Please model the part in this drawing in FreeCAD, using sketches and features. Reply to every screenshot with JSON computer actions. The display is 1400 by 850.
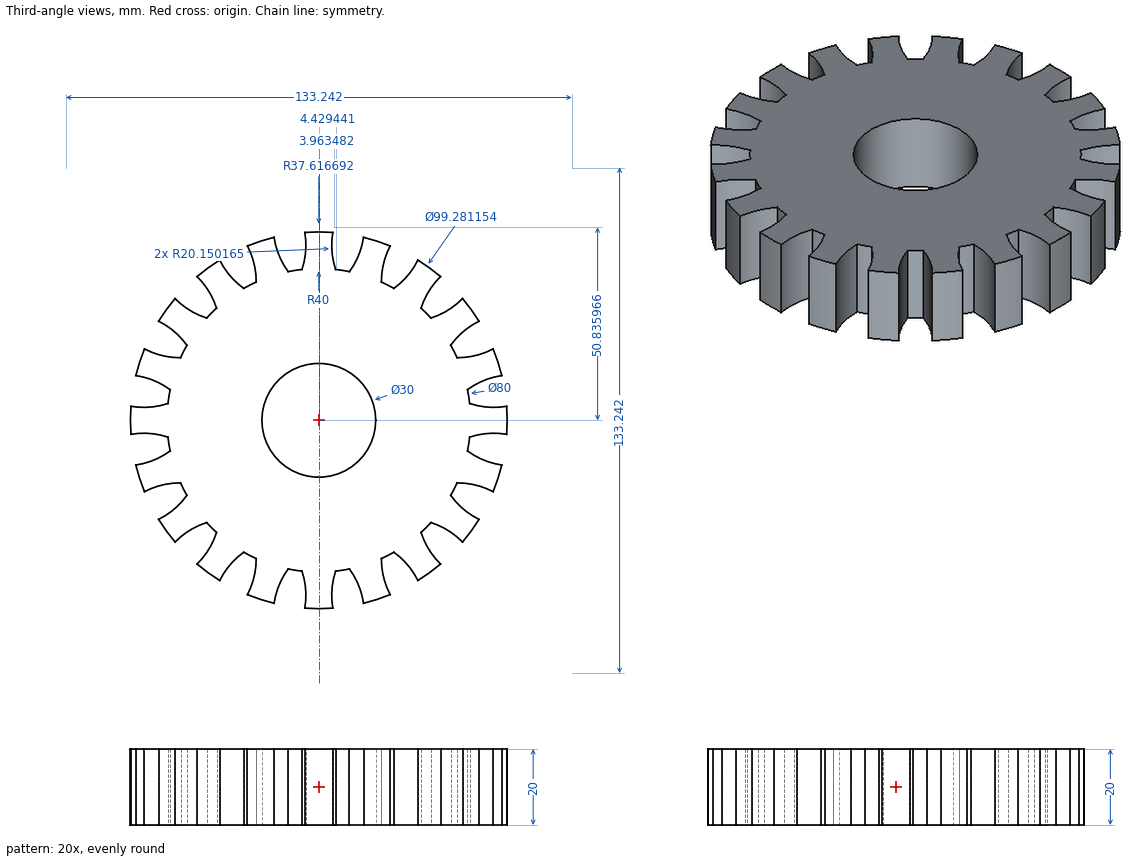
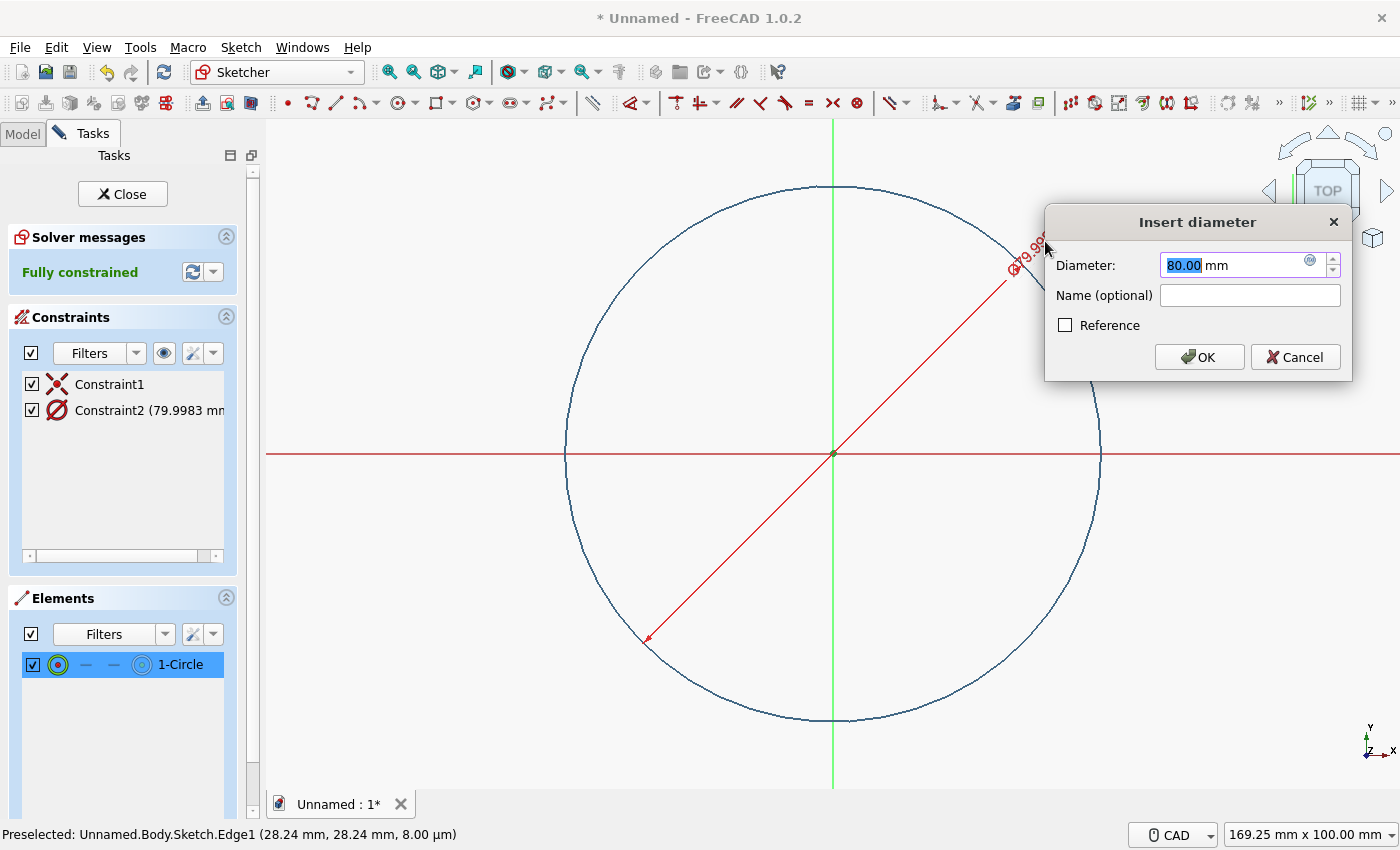
{"action": "type", "text": "80"}
{"action": "key", "text": "Return"}
{"action": "key", "text": "Escape"}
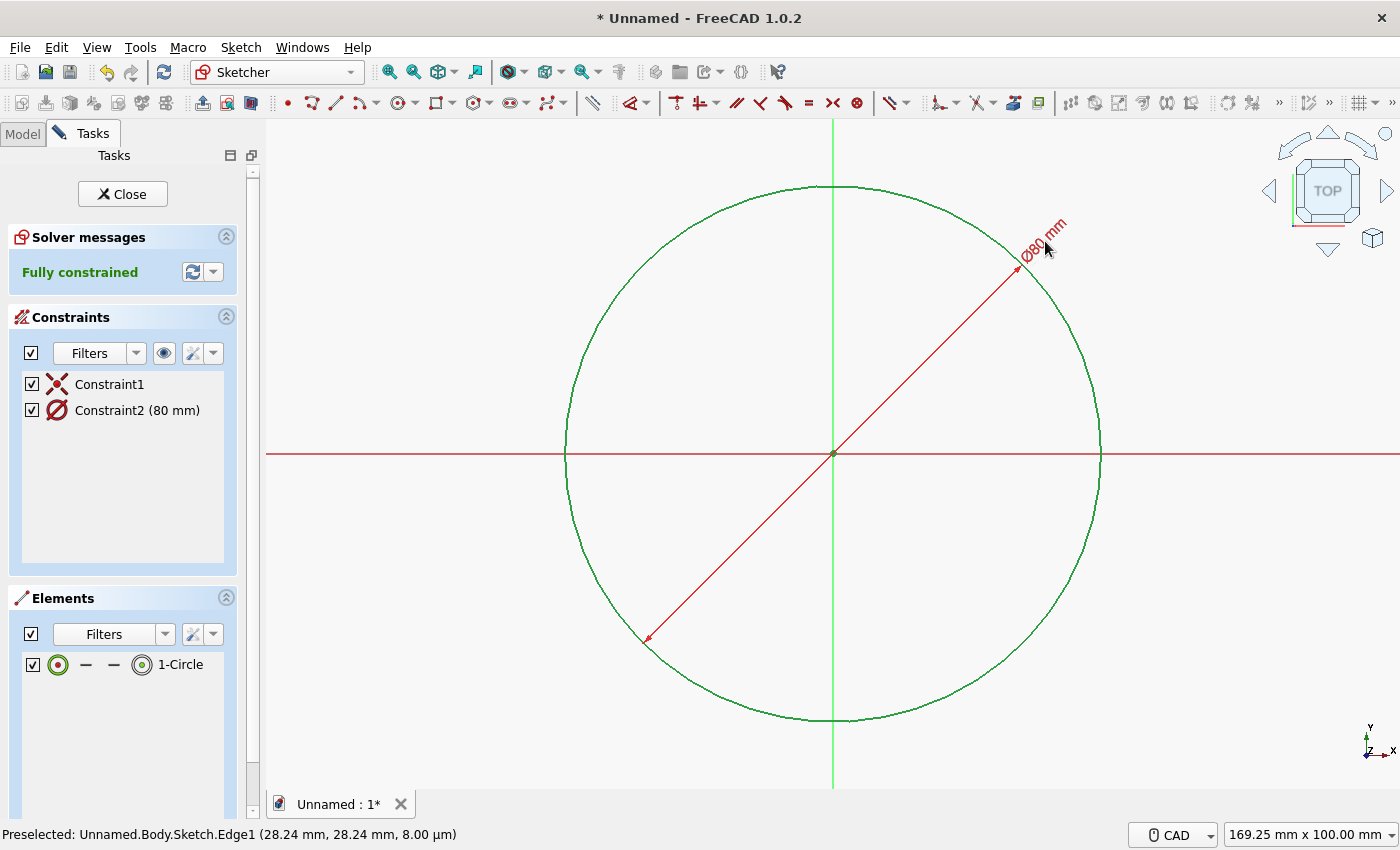
{"action": "left_click", "coordinate": [123, 194]}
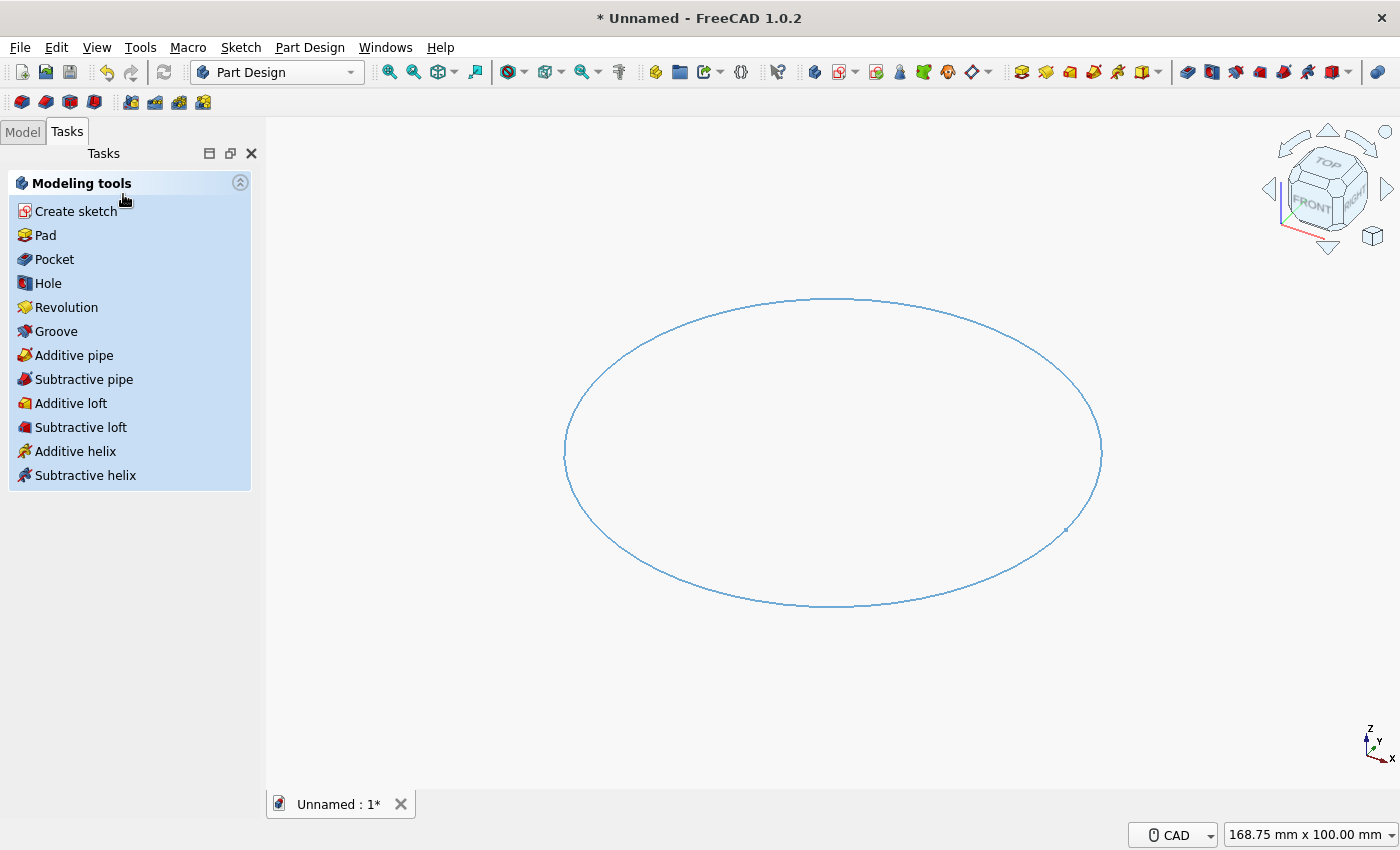
{"action": "left_click", "coordinate": [1022, 72]}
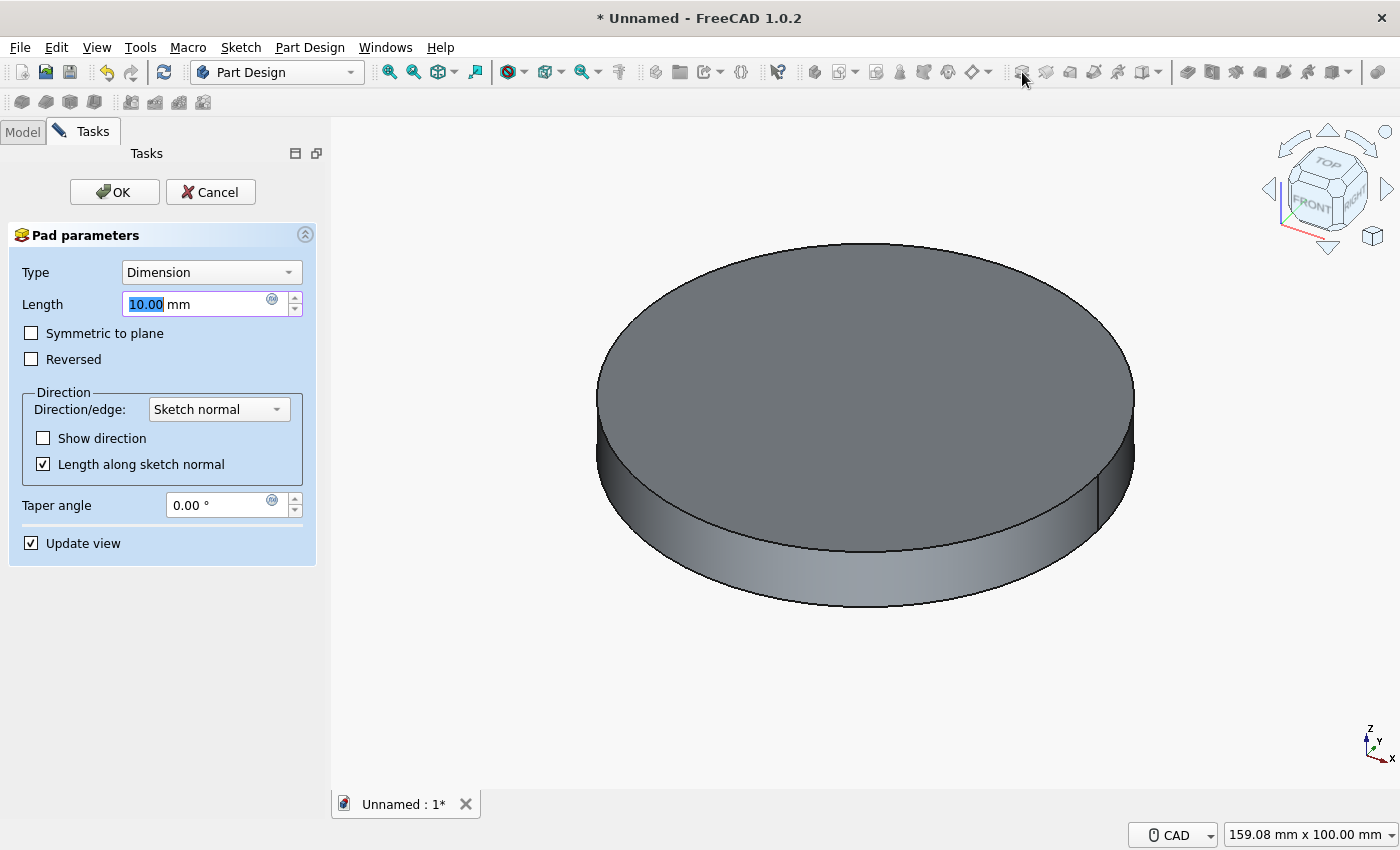
{"action": "type", "text": "20"}
{"action": "key", "text": "Tab"}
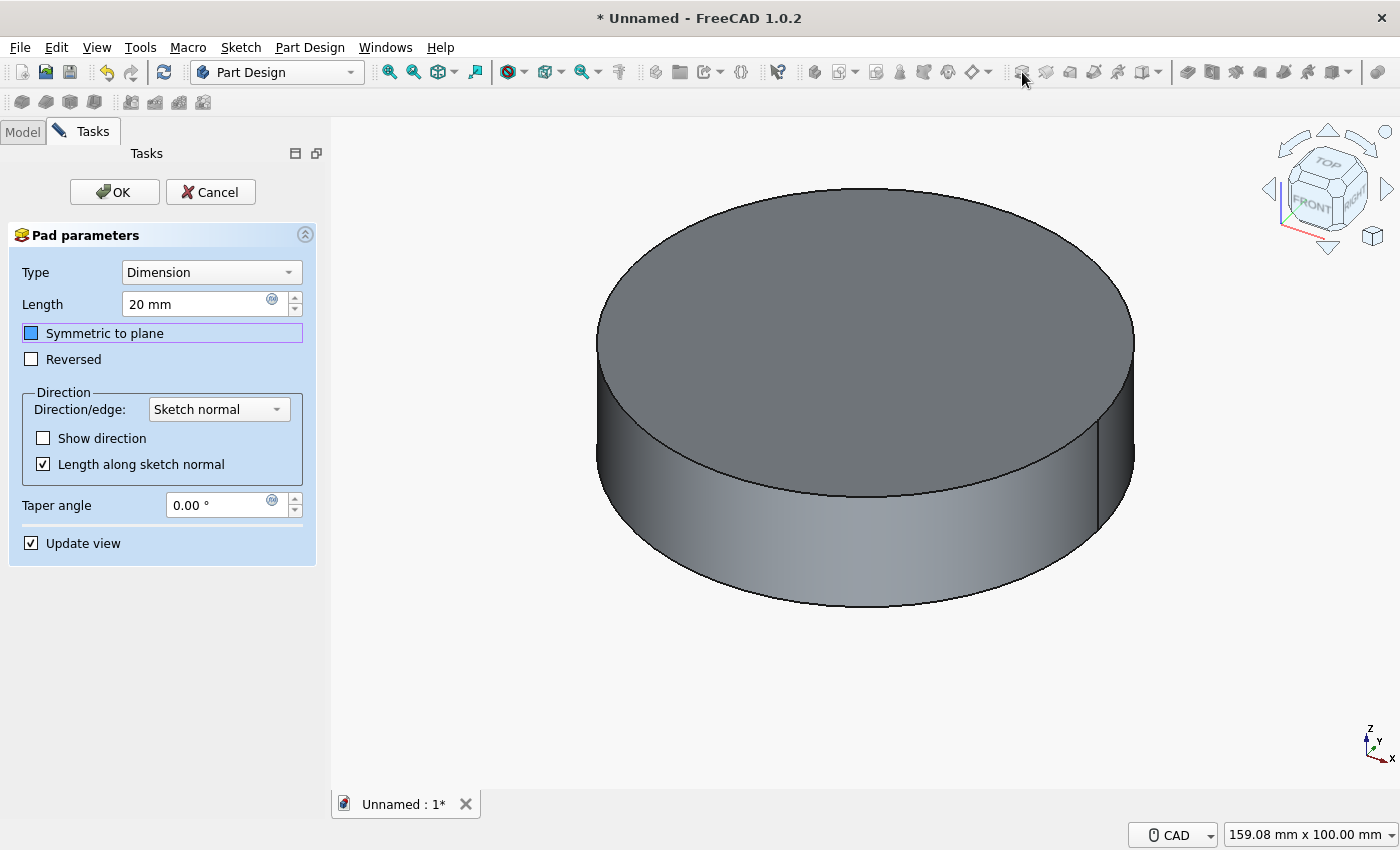
{"action": "left_click", "coordinate": [30, 333]}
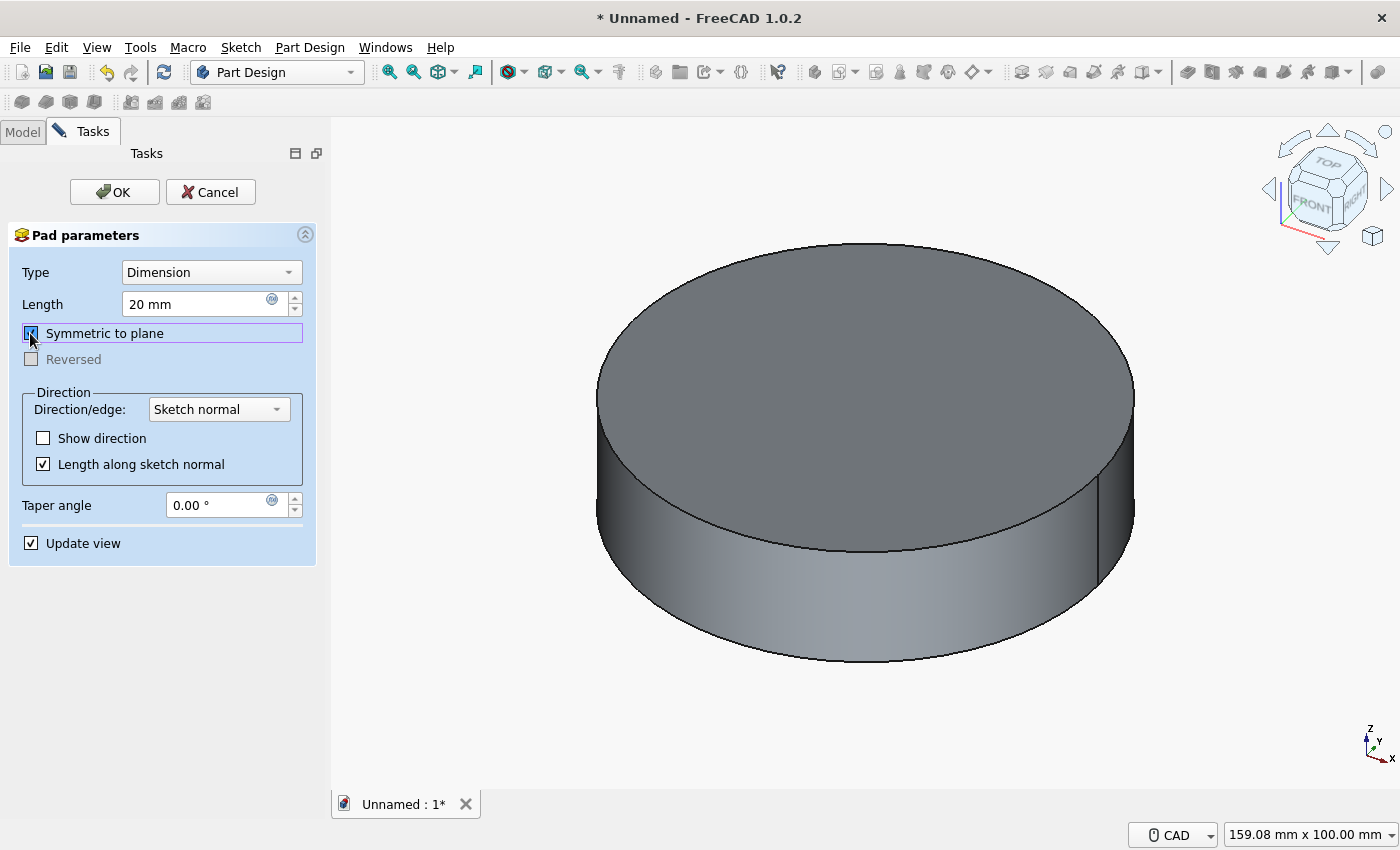
{"action": "left_click", "coordinate": [115, 192]}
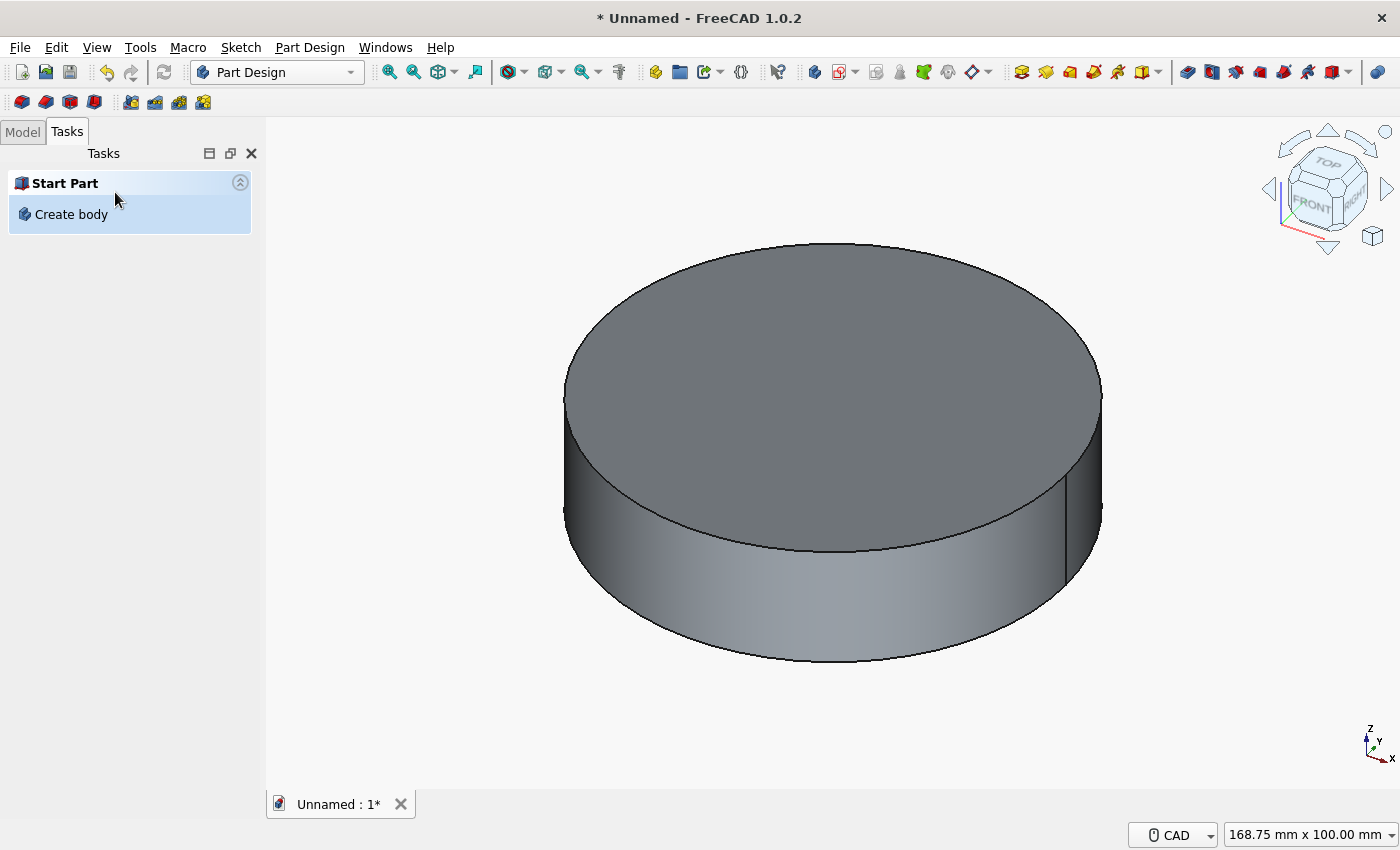
{"action": "left_click", "coordinate": [833, 397]}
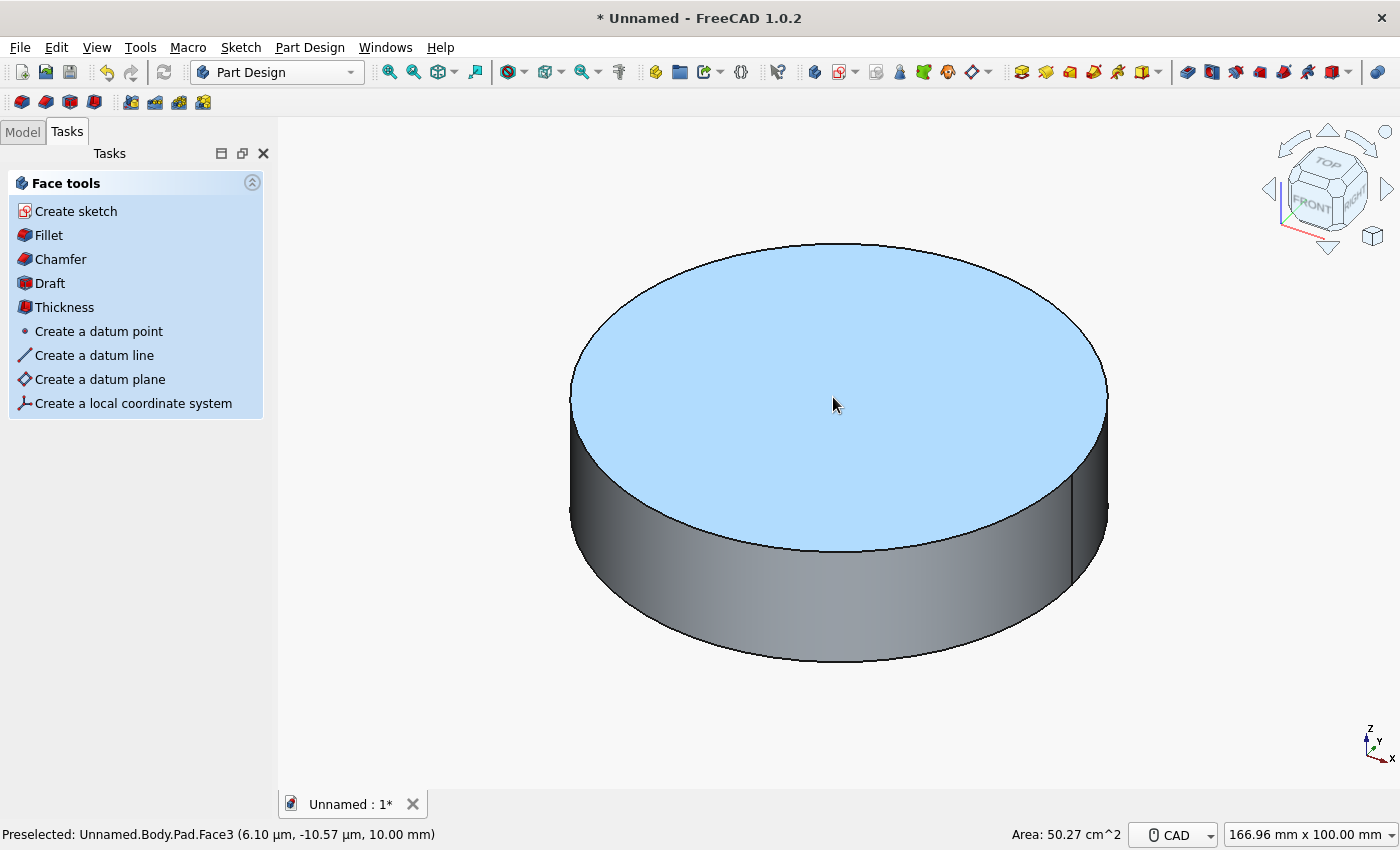
{"action": "left_click", "coordinate": [840, 72]}